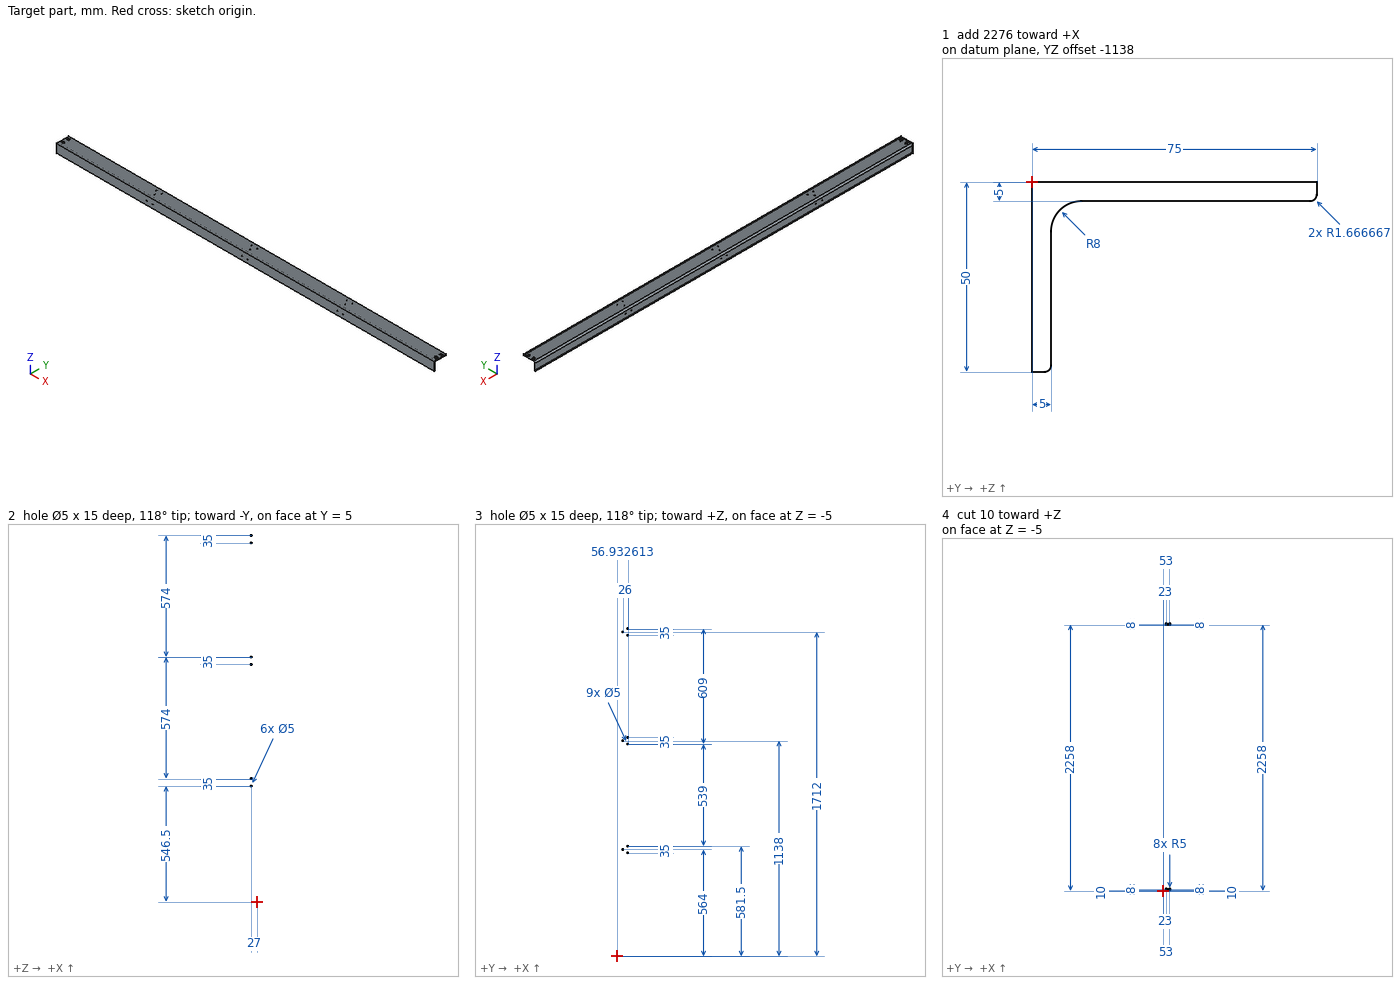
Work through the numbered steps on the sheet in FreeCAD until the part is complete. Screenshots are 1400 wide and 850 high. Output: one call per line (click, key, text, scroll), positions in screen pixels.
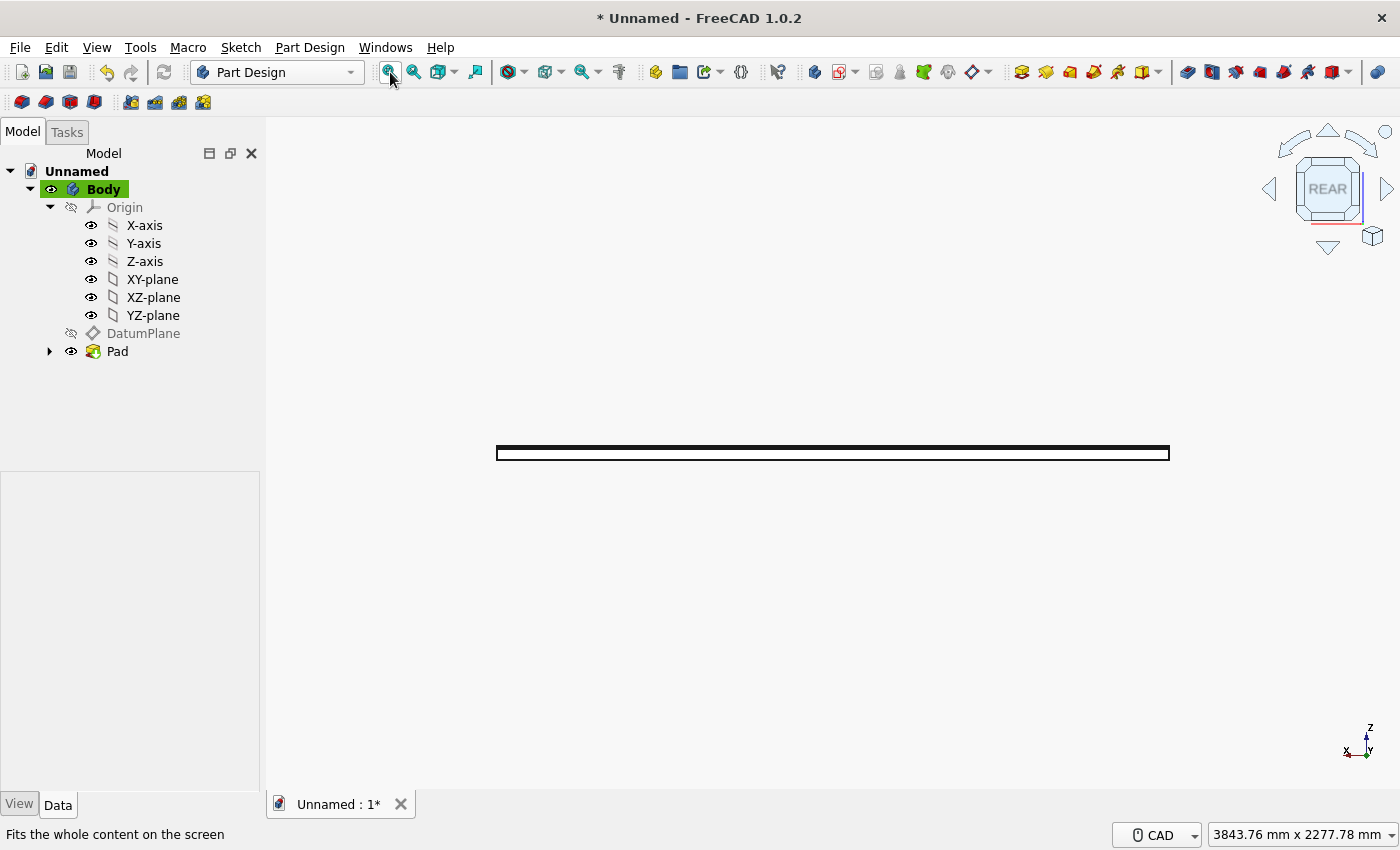
scroll(833, 454, up, 5)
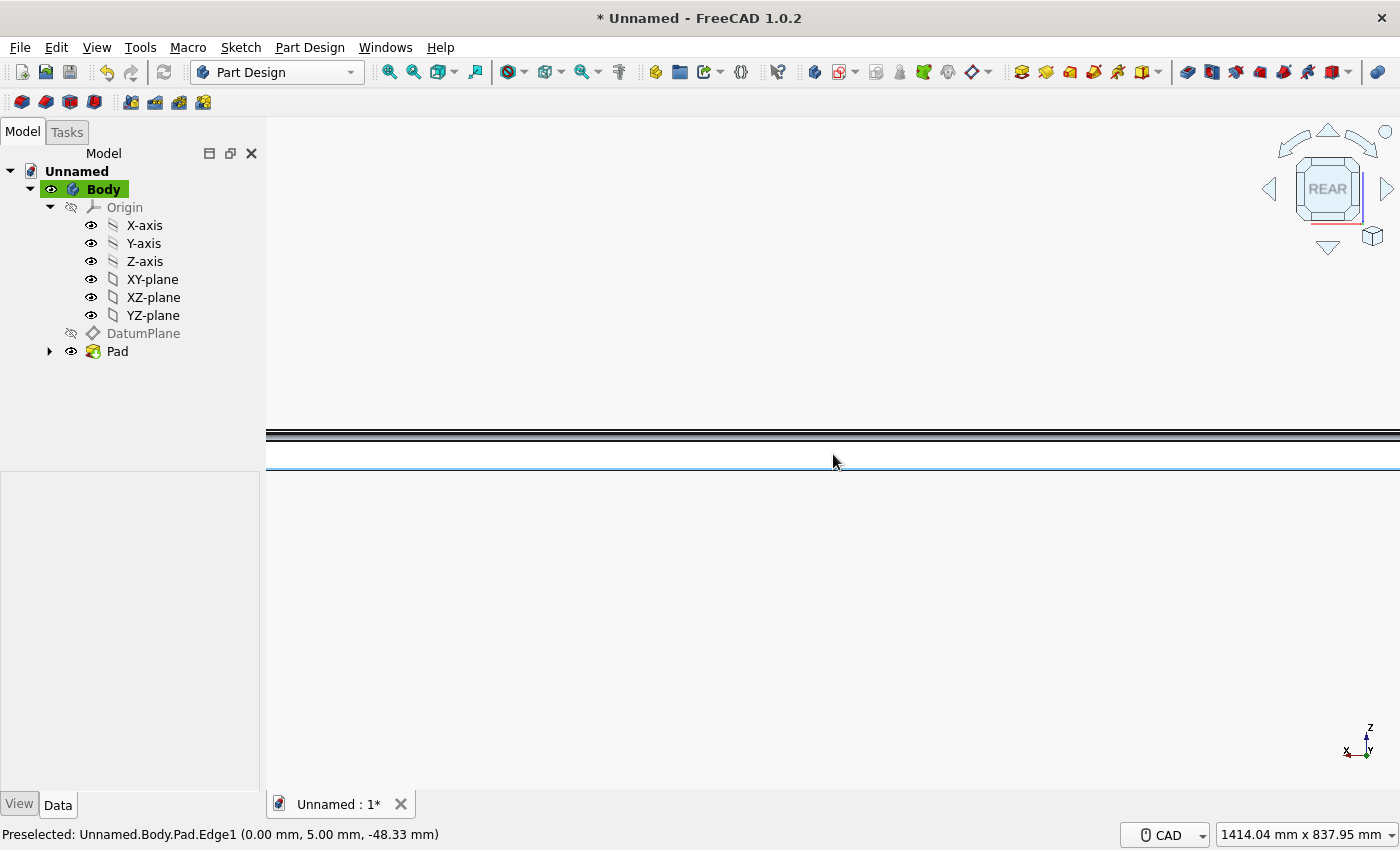
click(832, 454)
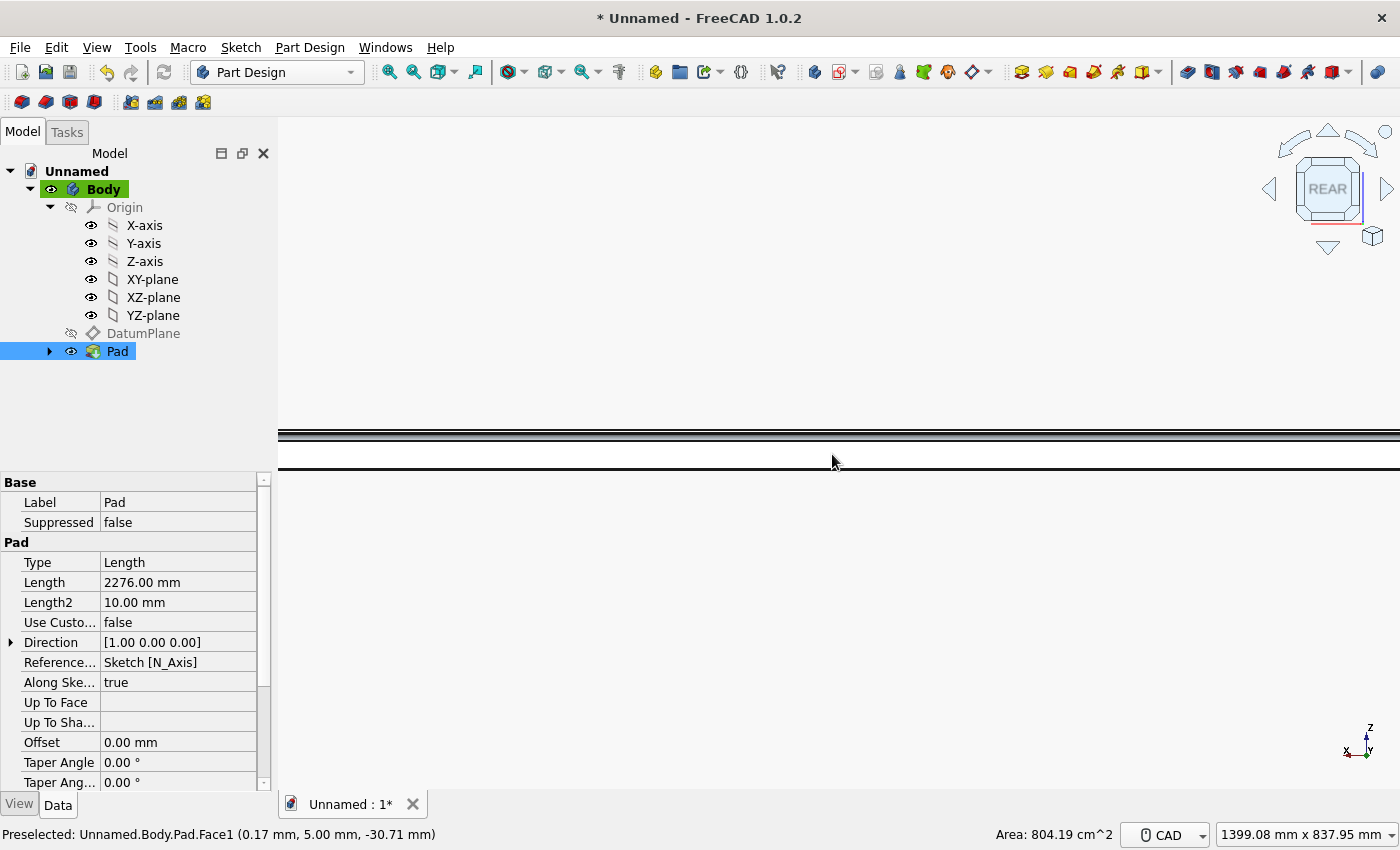
click(840, 72)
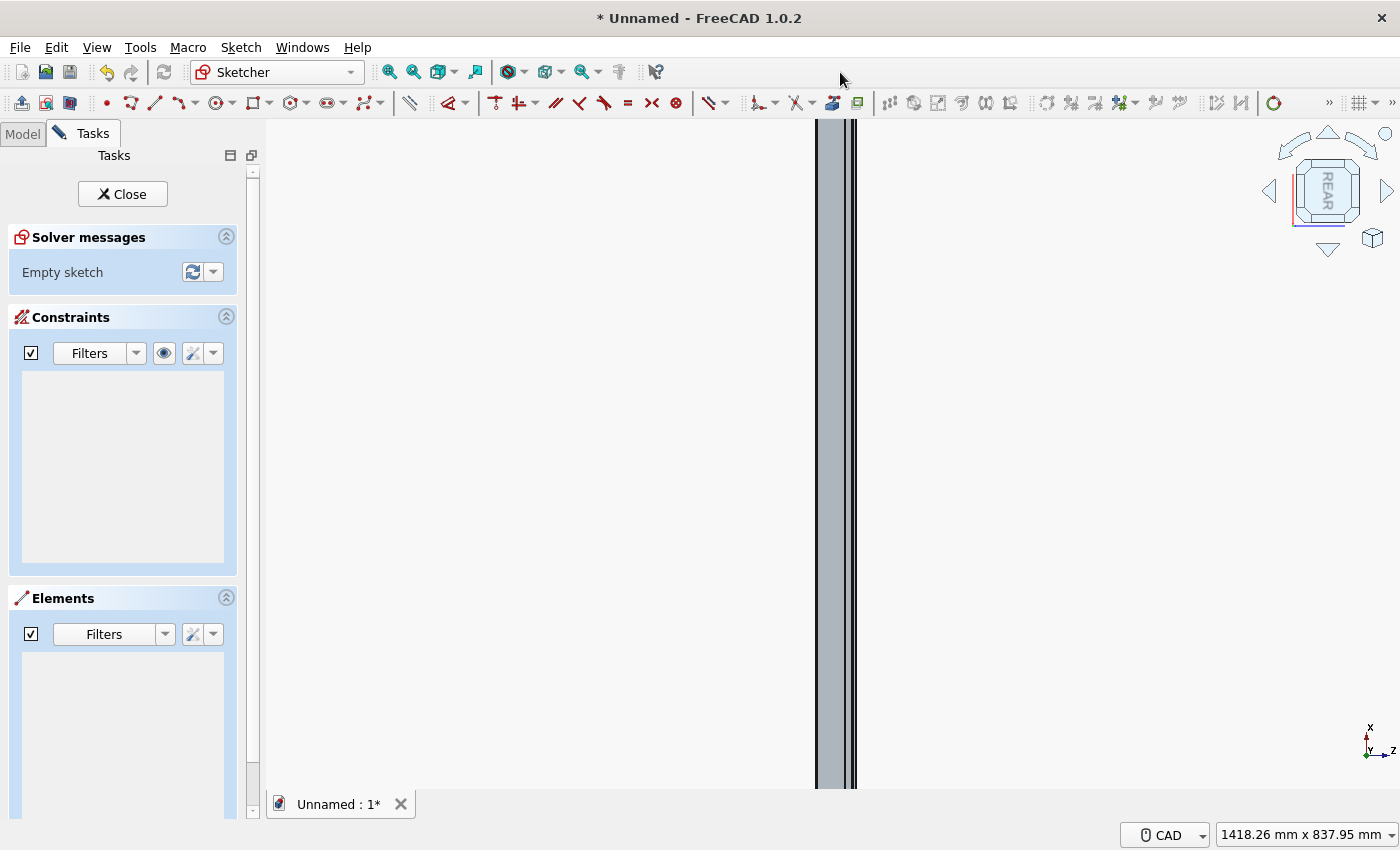
scroll(730, 361, down, 6)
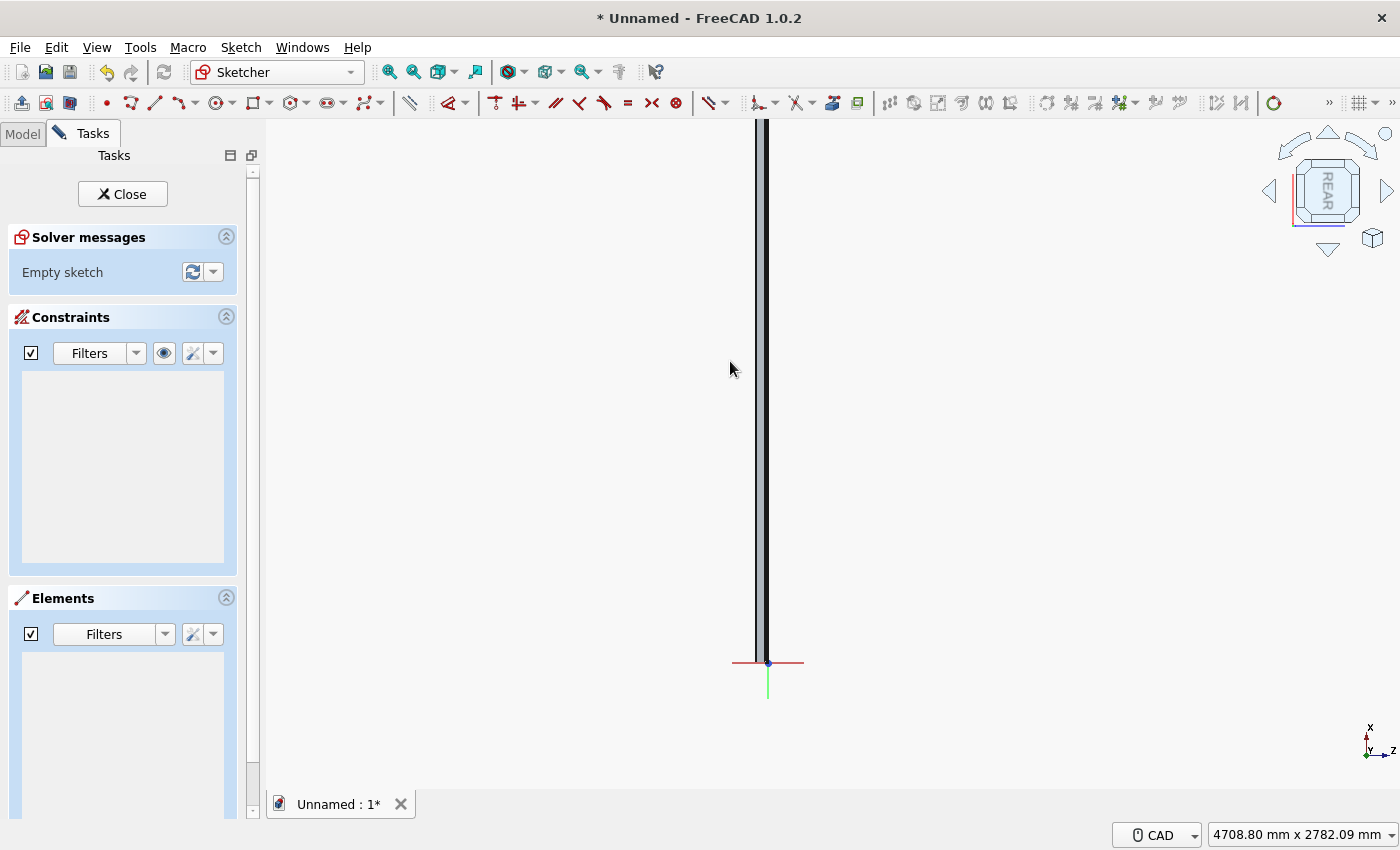
click(216, 104)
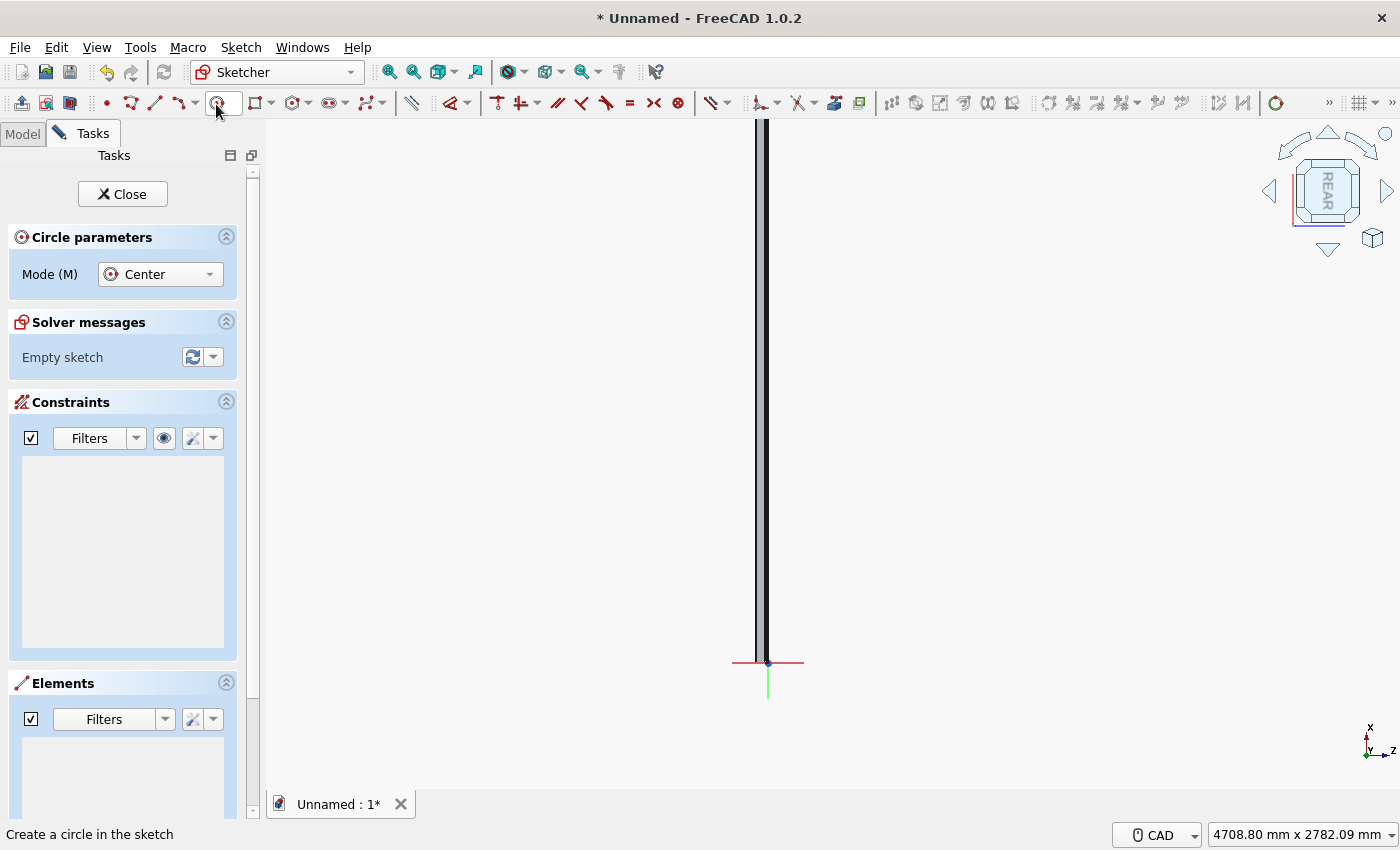
scroll(762, 531, up, 19)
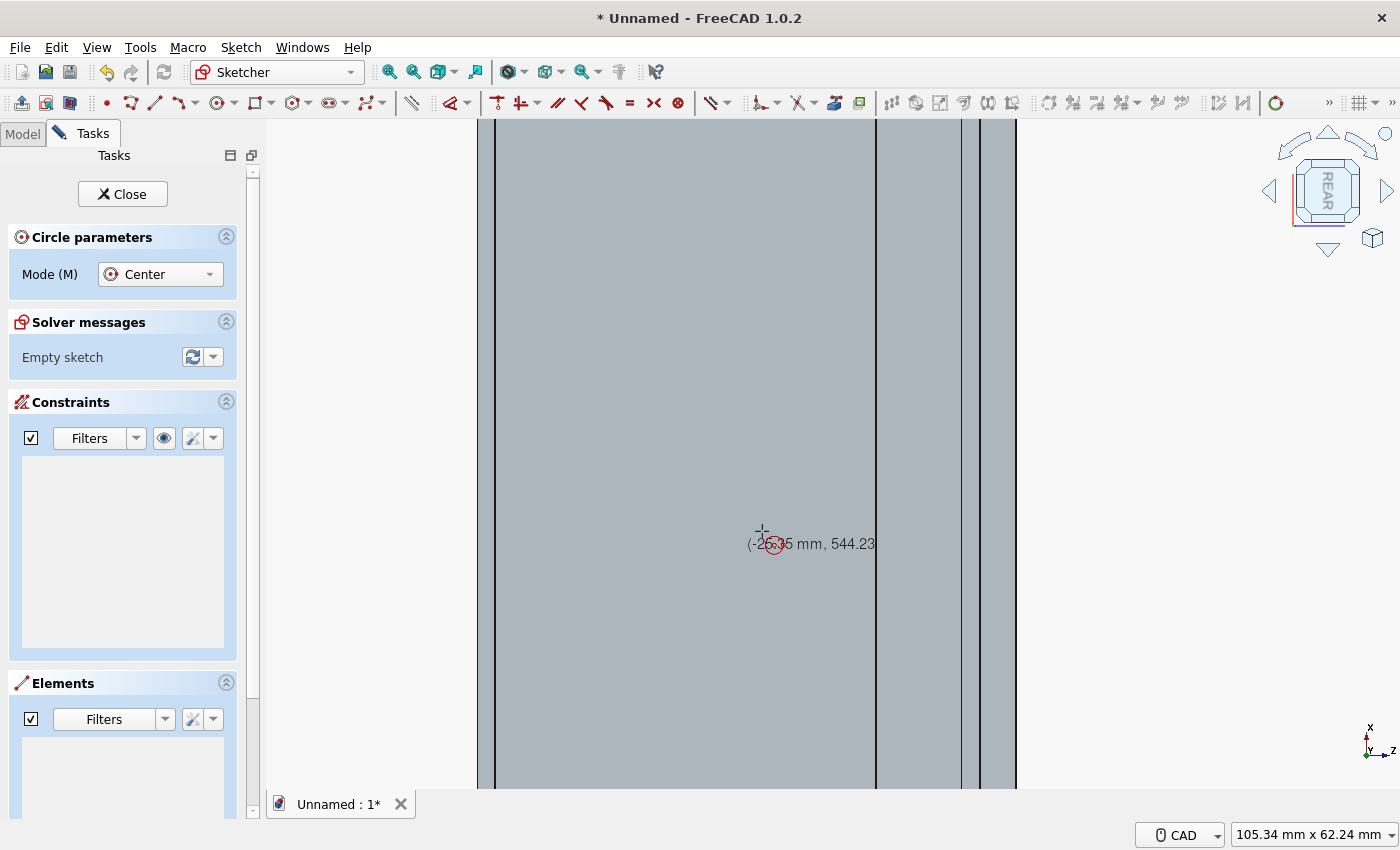
scroll(762, 549, down, 18)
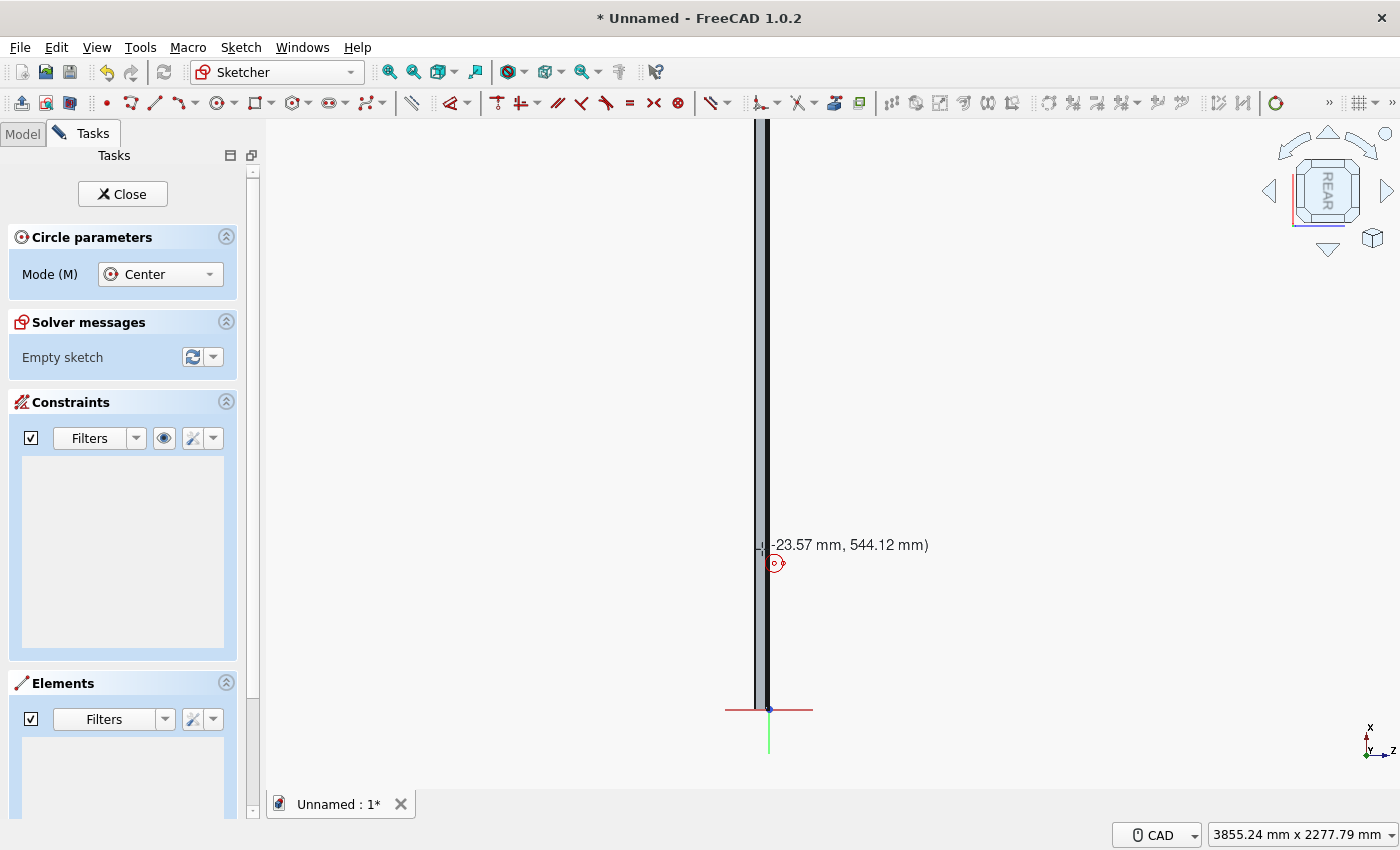
scroll(761, 549, up, 4)